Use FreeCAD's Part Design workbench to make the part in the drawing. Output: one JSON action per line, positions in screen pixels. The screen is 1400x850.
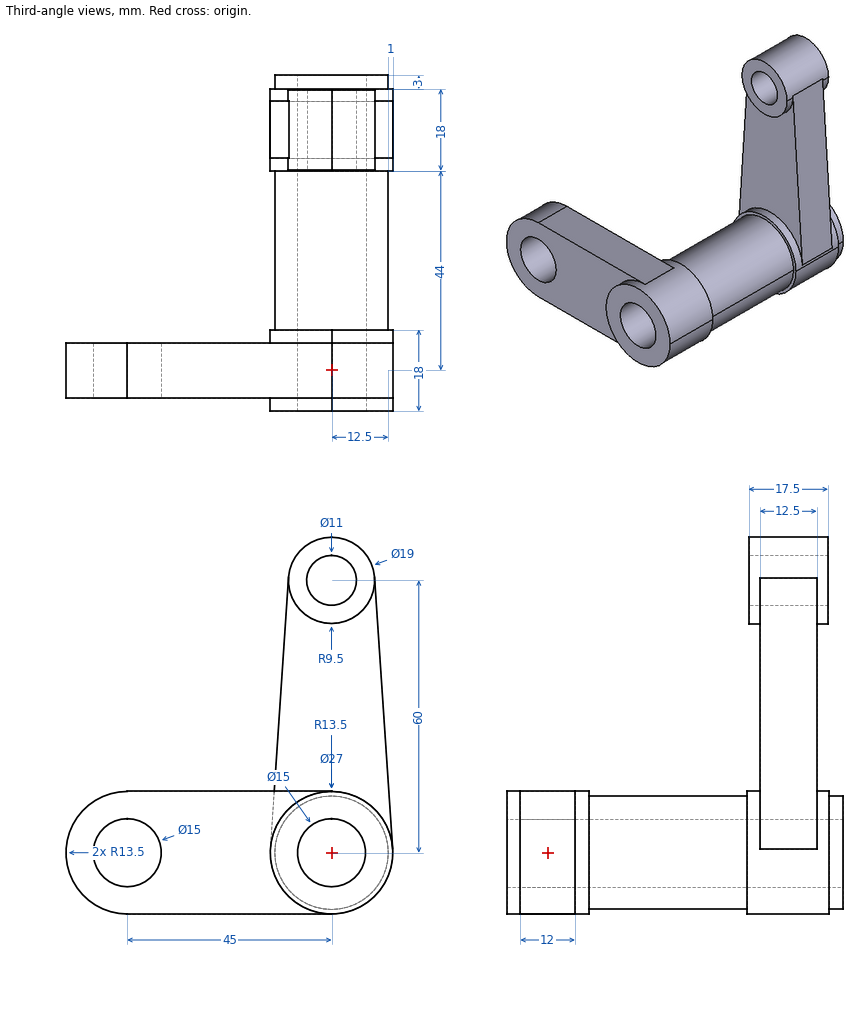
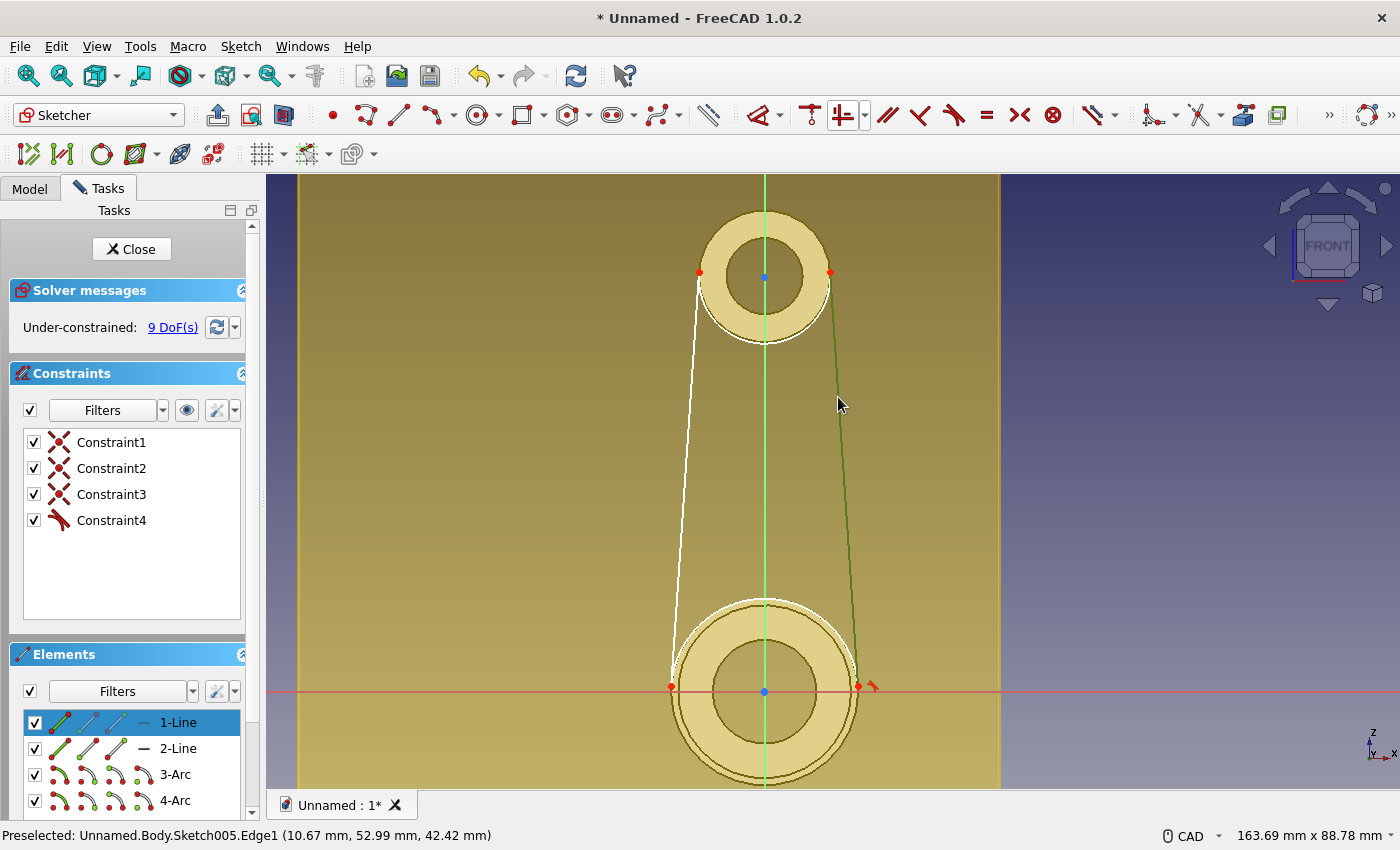
{"action": "left_click", "coordinate": [724, 330]}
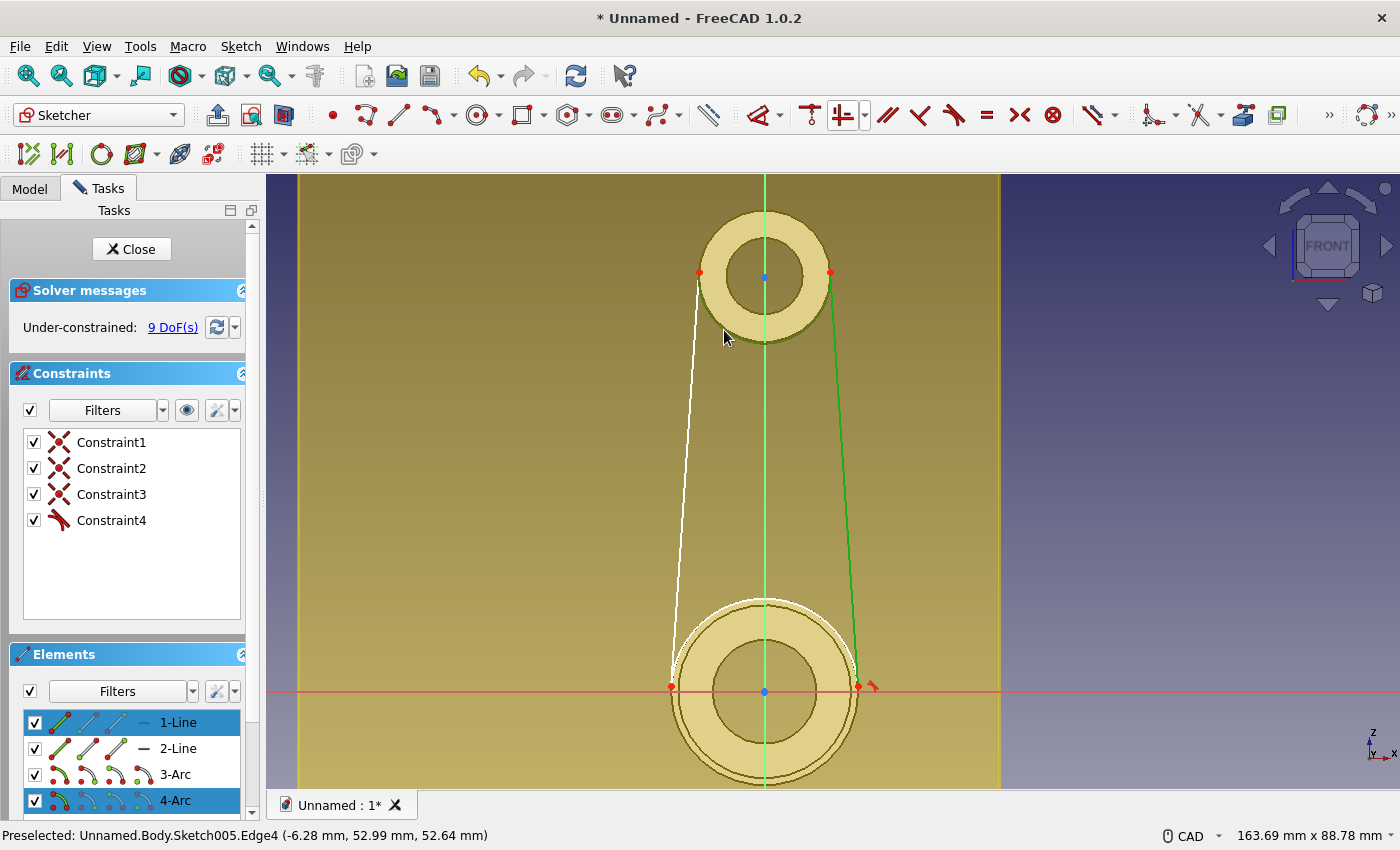
{"action": "left_click", "coordinate": [954, 116]}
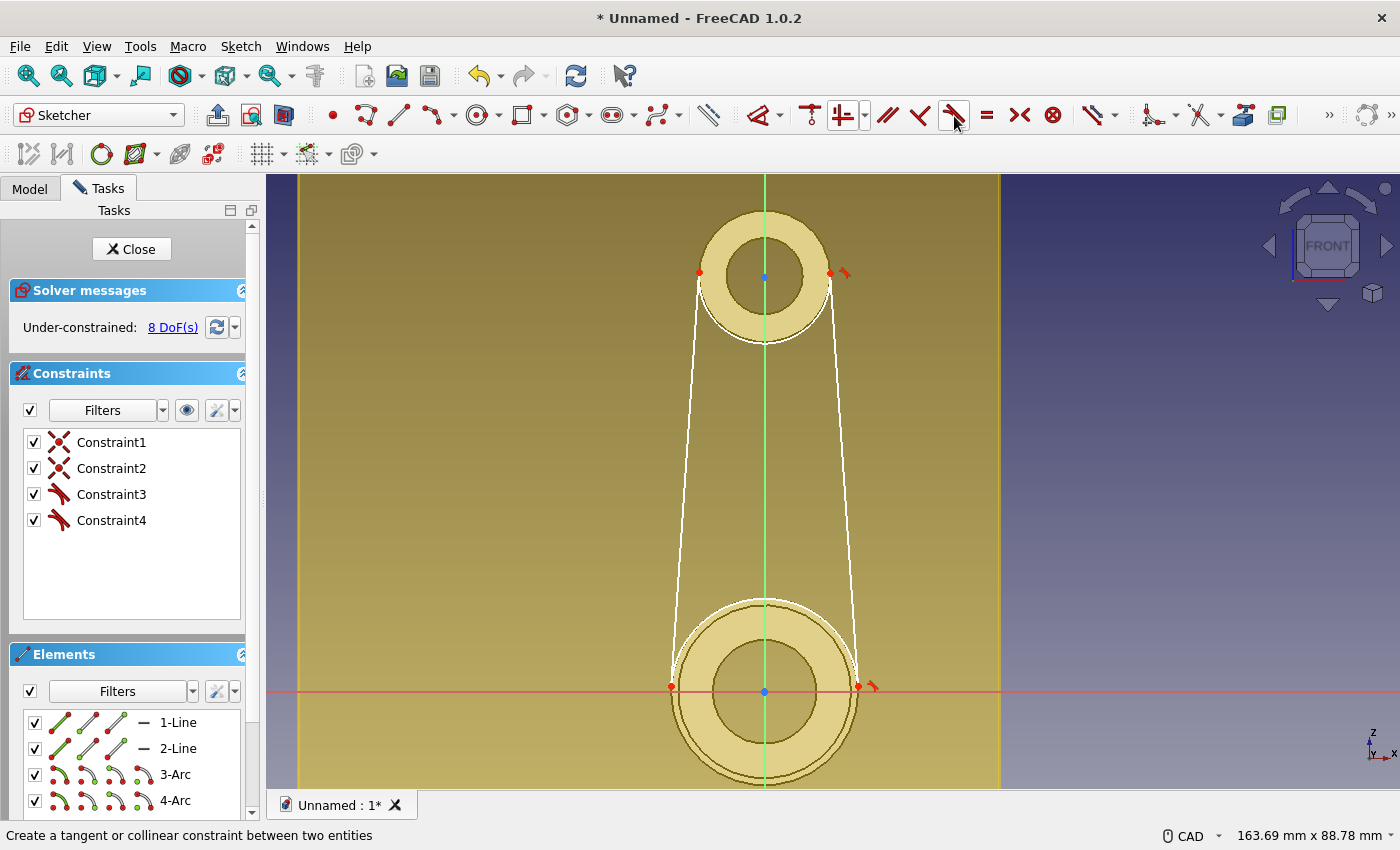
{"action": "left_click", "coordinate": [680, 562]}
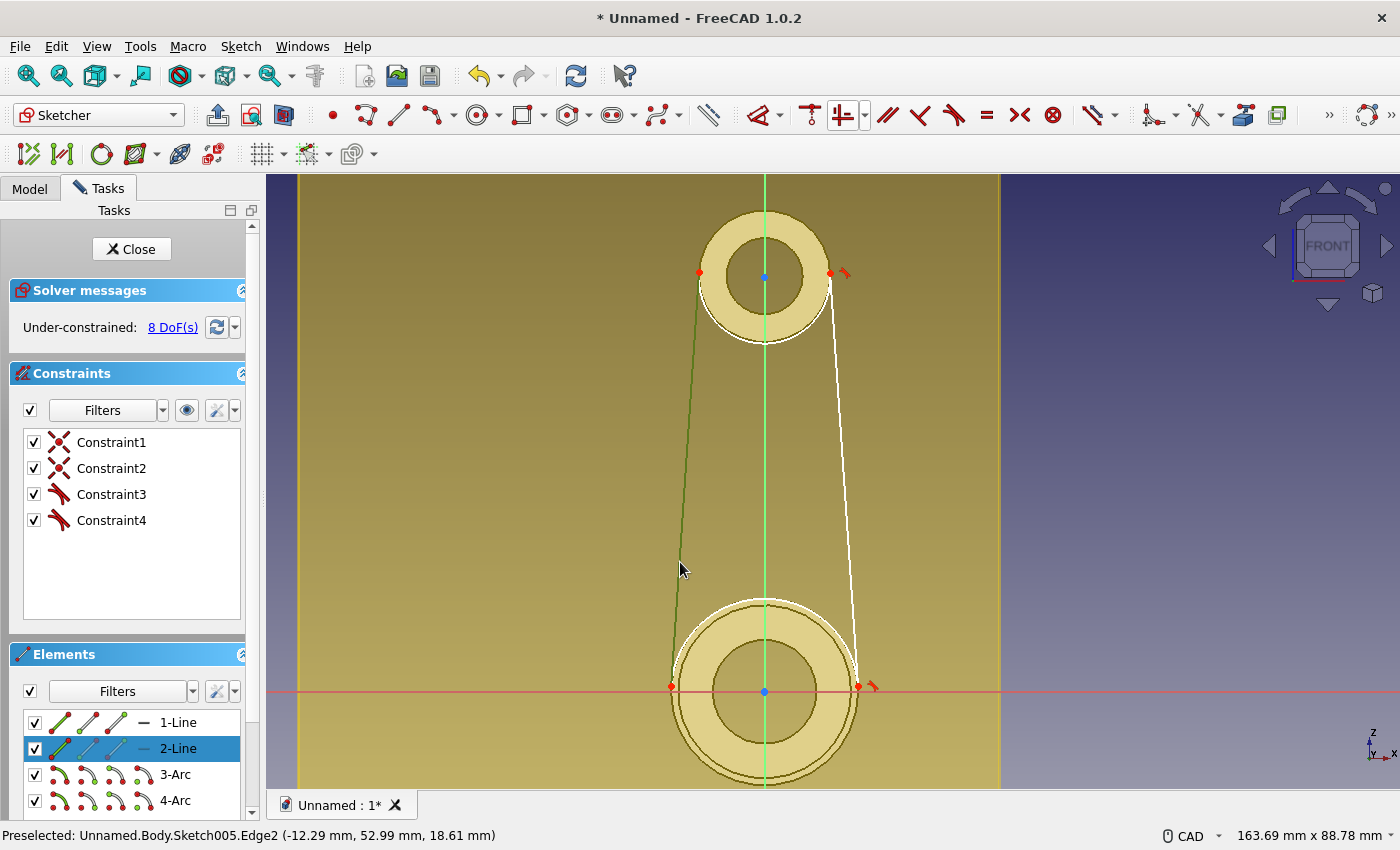
{"action": "left_click", "coordinate": [818, 615]}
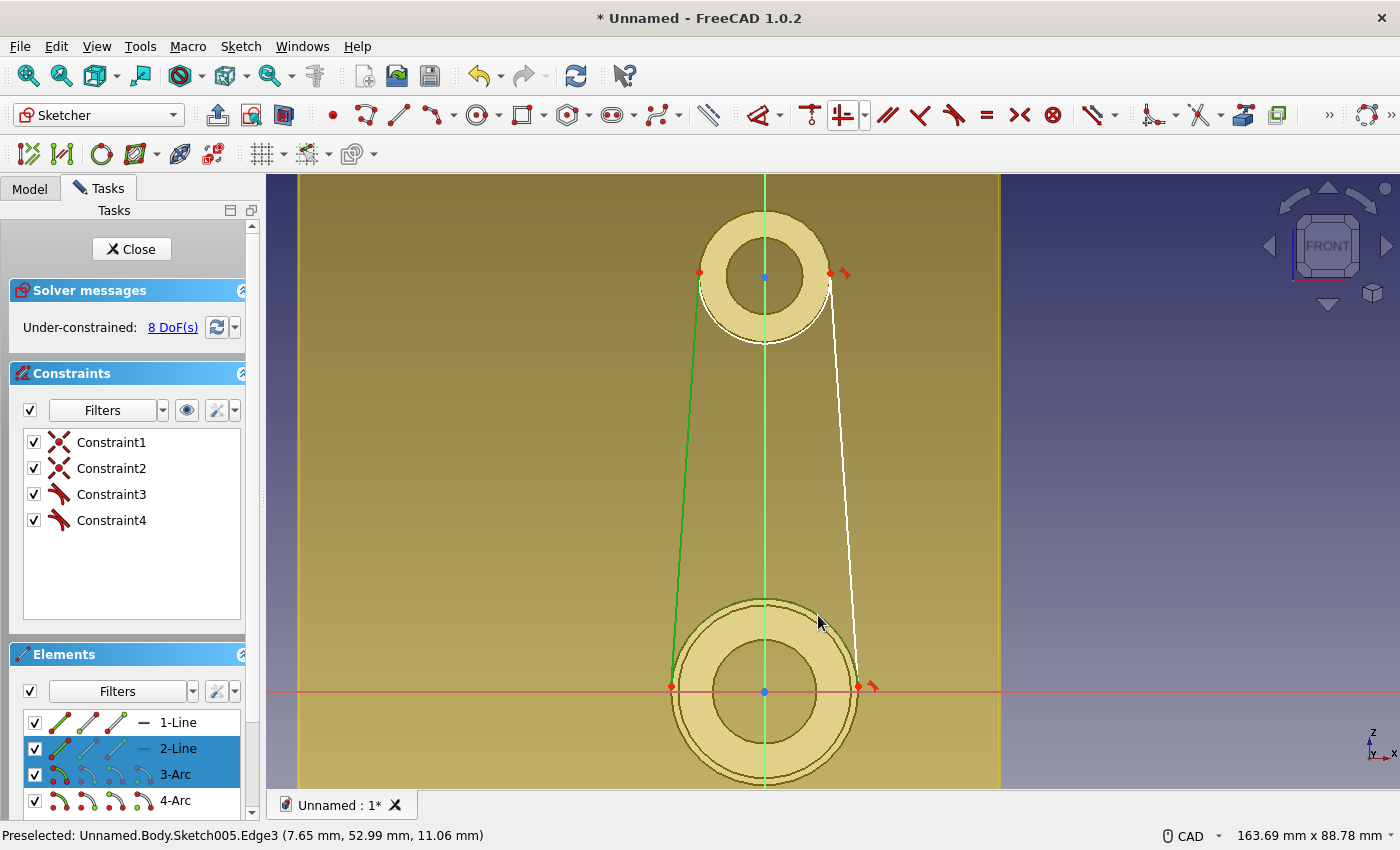
{"action": "left_click", "coordinate": [954, 116]}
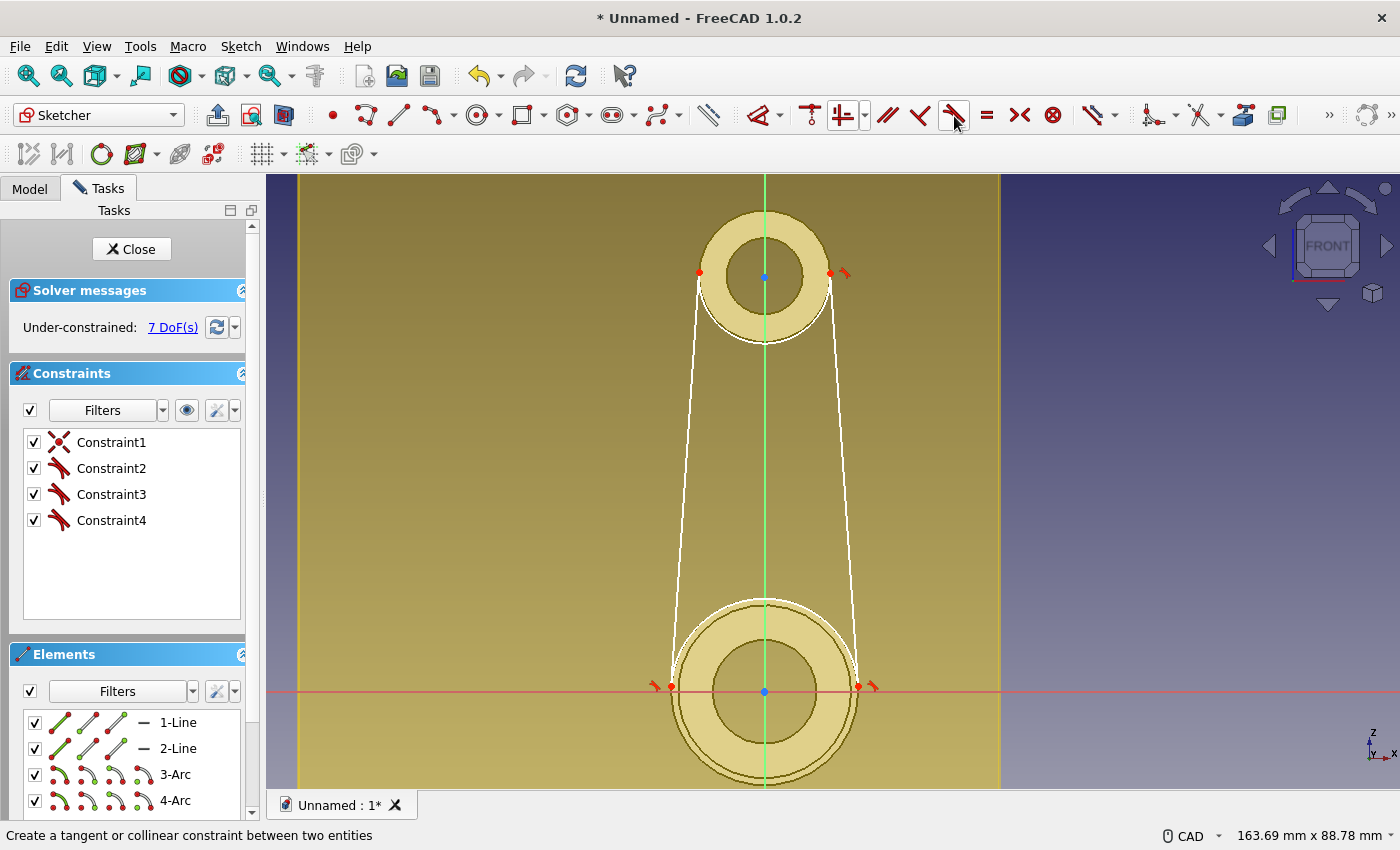
{"action": "left_click", "coordinate": [680, 562]}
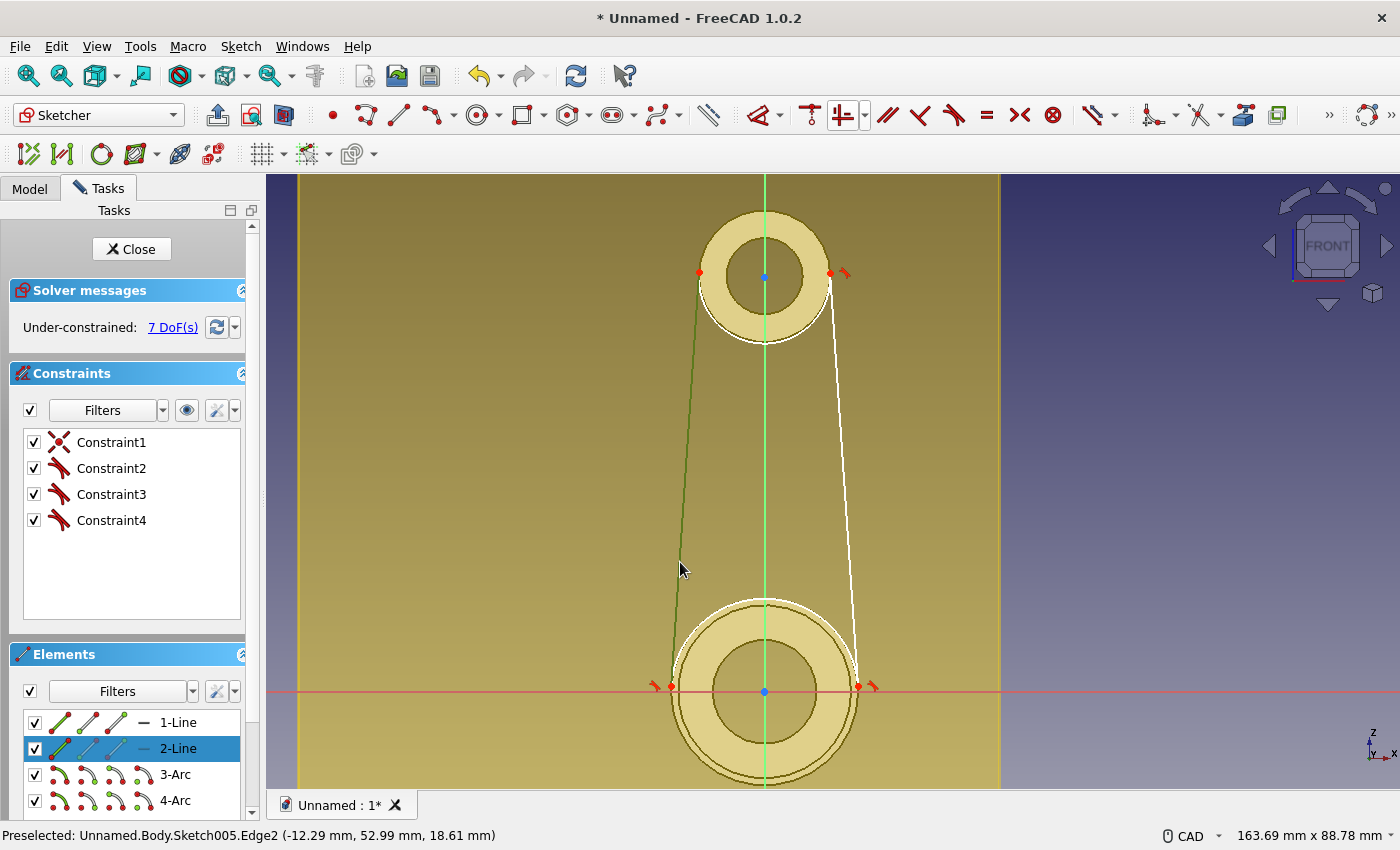
{"action": "left_click", "coordinate": [724, 330]}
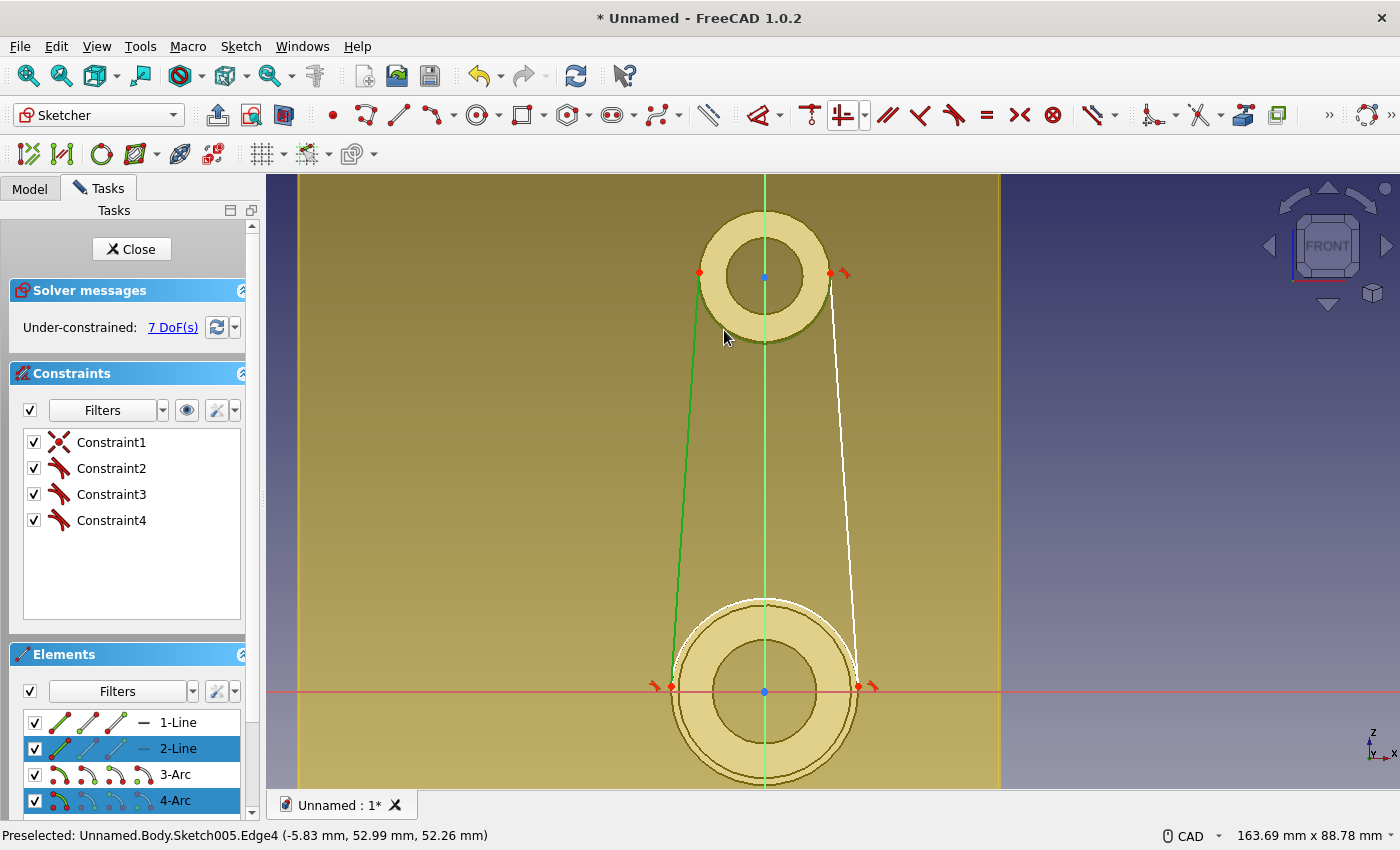
{"action": "key", "text": "t"}